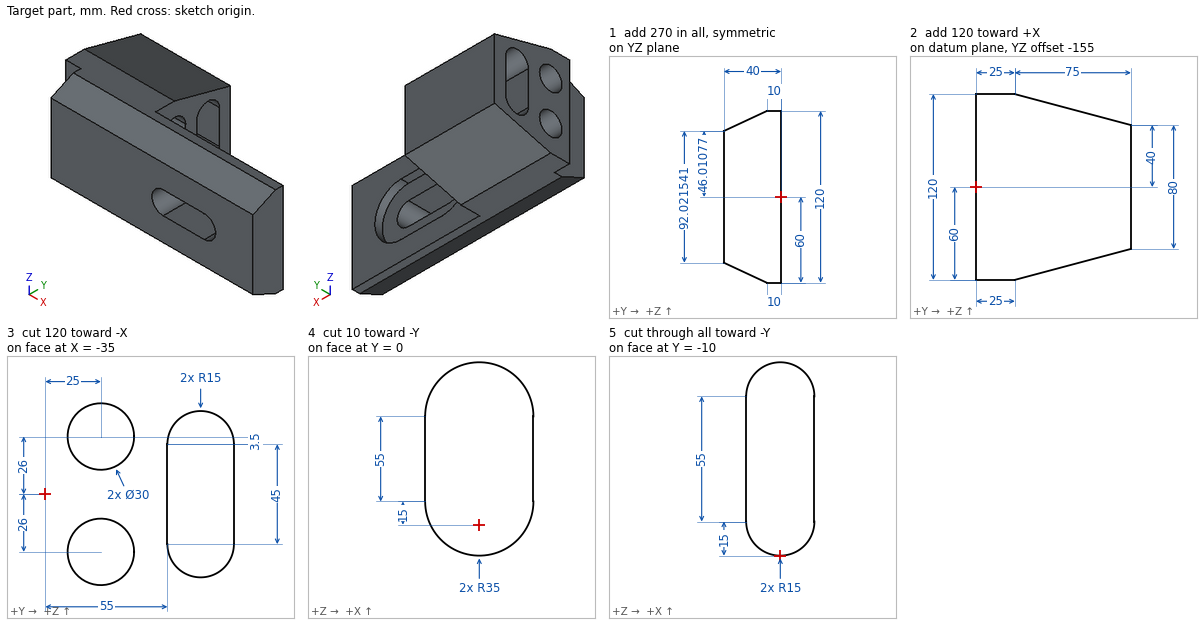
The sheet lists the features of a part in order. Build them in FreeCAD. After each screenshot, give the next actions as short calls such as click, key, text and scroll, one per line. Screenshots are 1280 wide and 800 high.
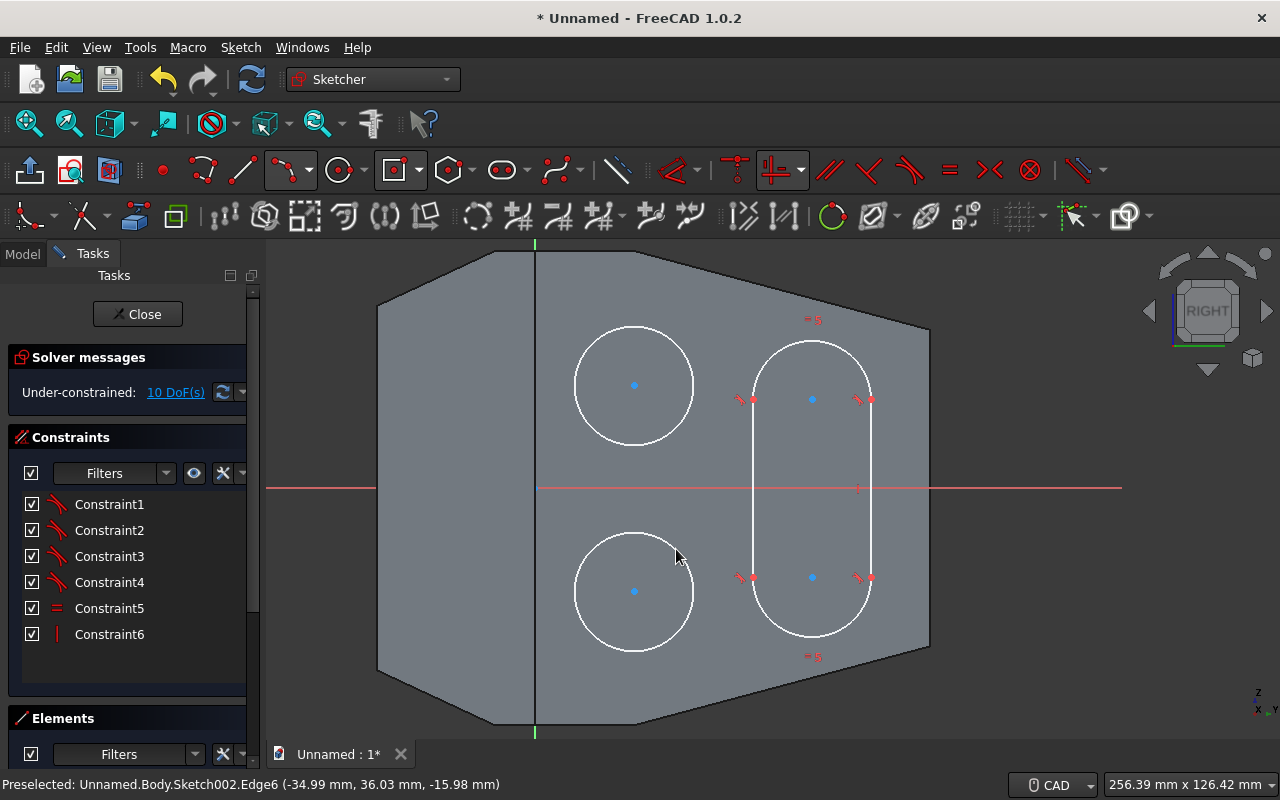
click(676, 344)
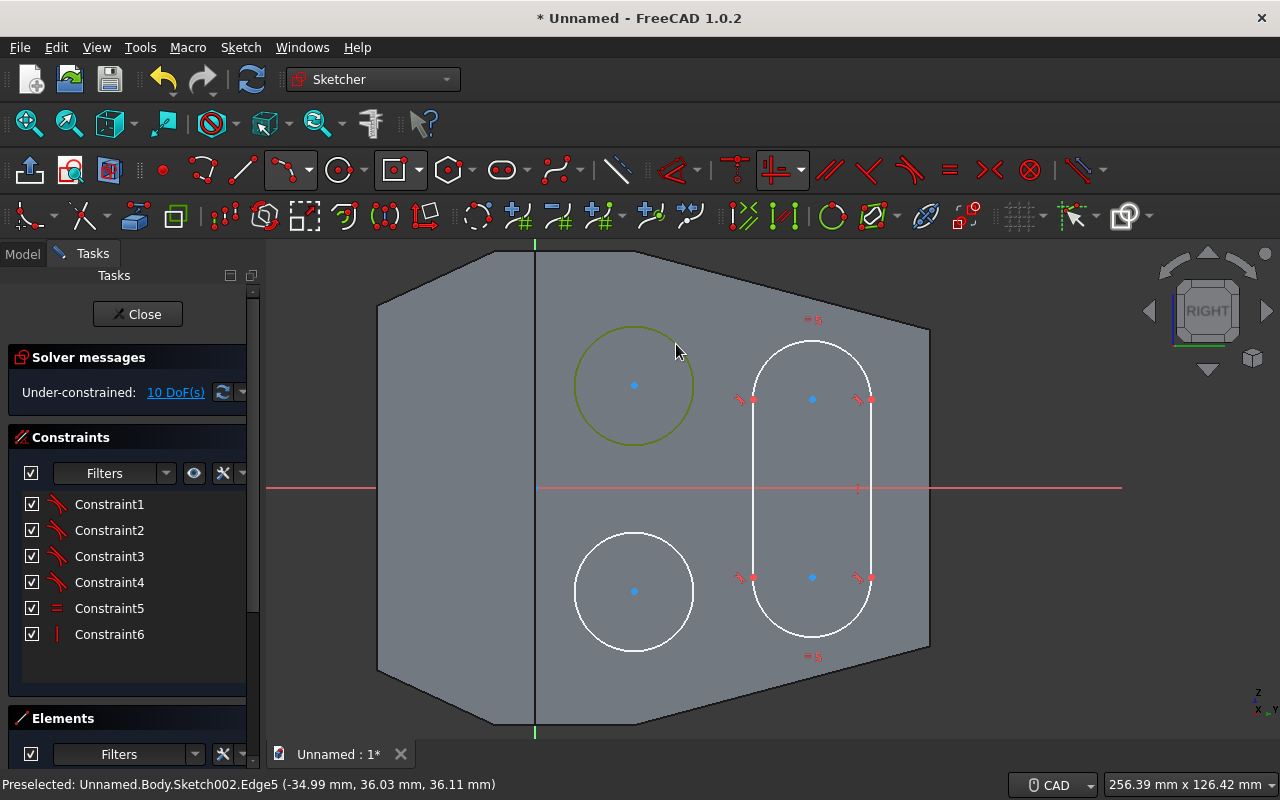
click(676, 550)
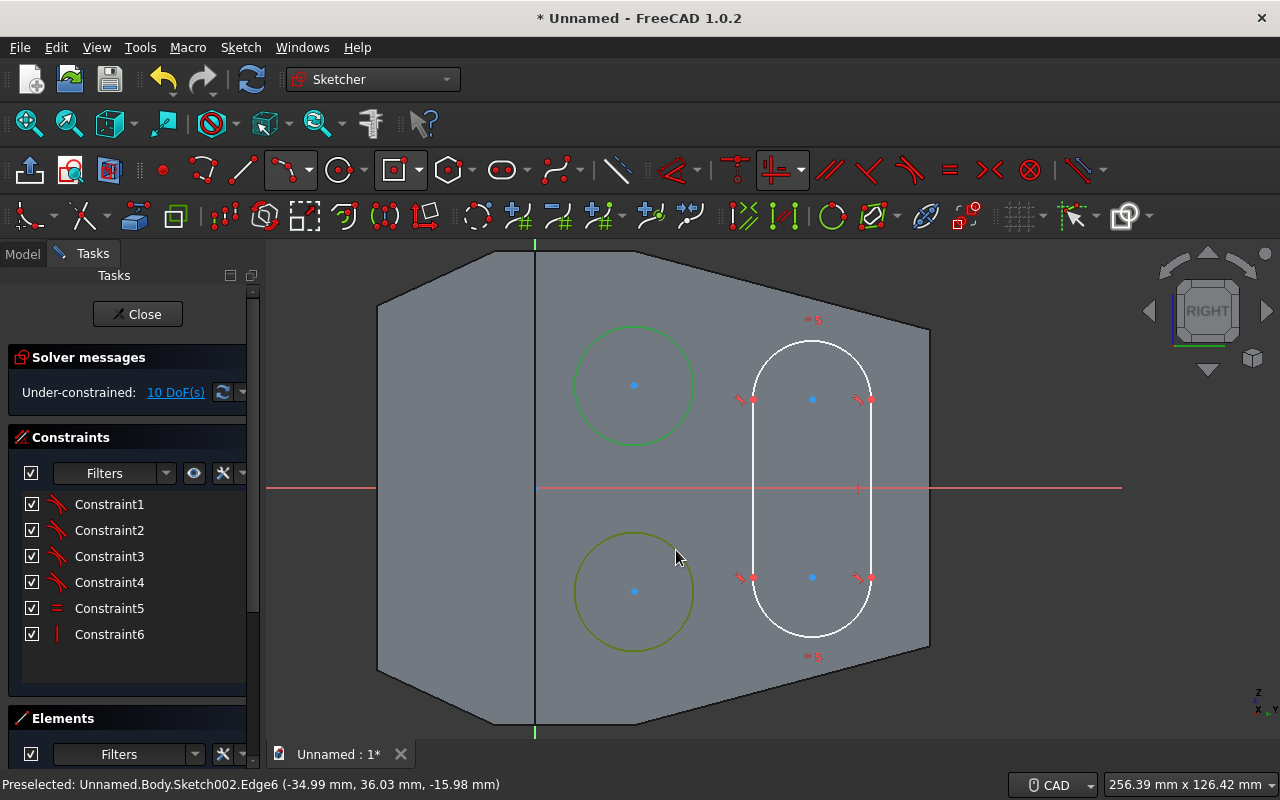
click(950, 170)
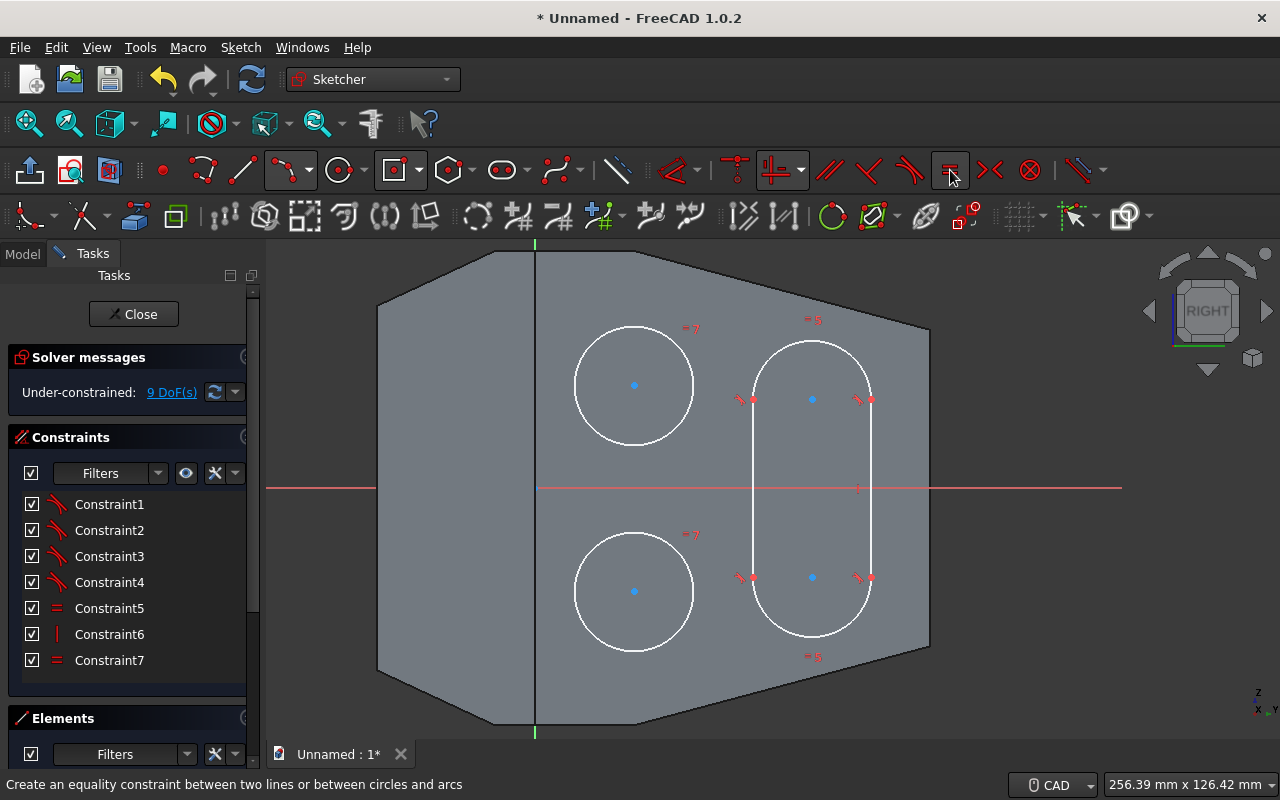
click(634, 386)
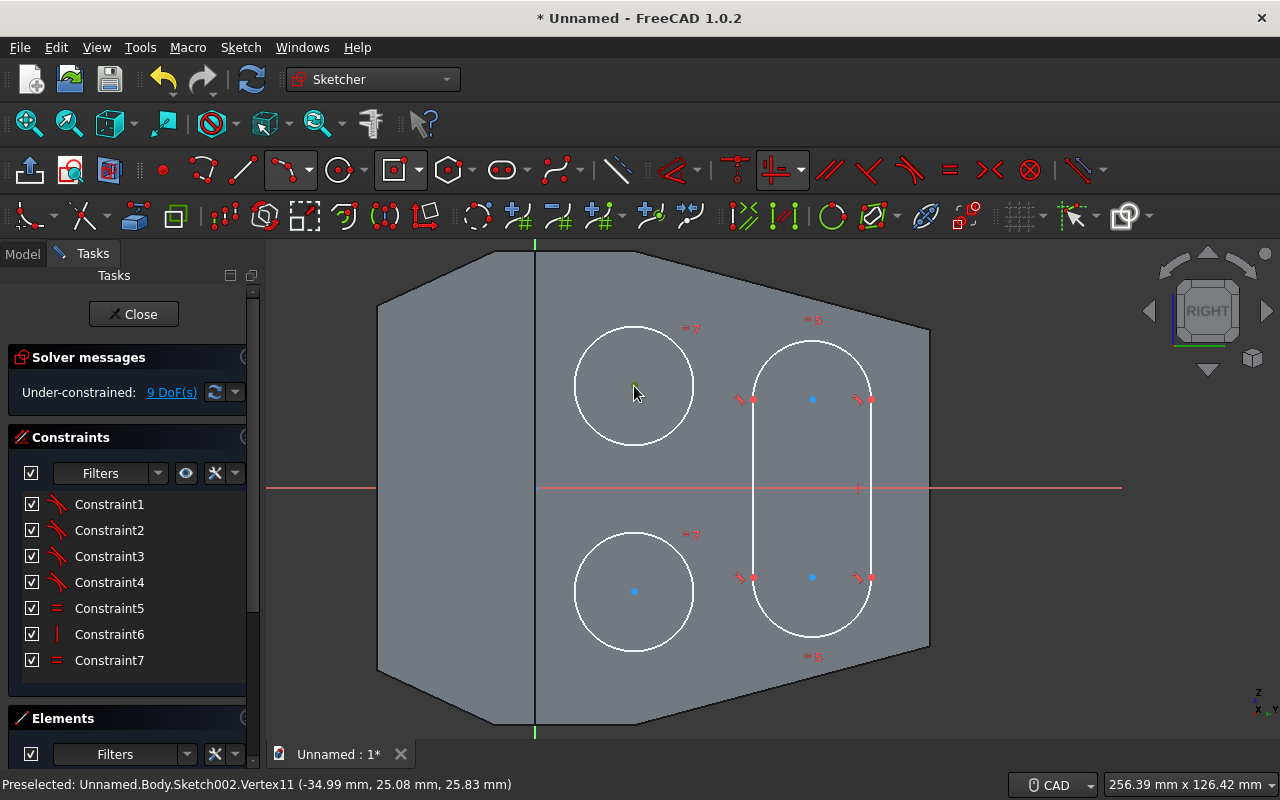
click(634, 592)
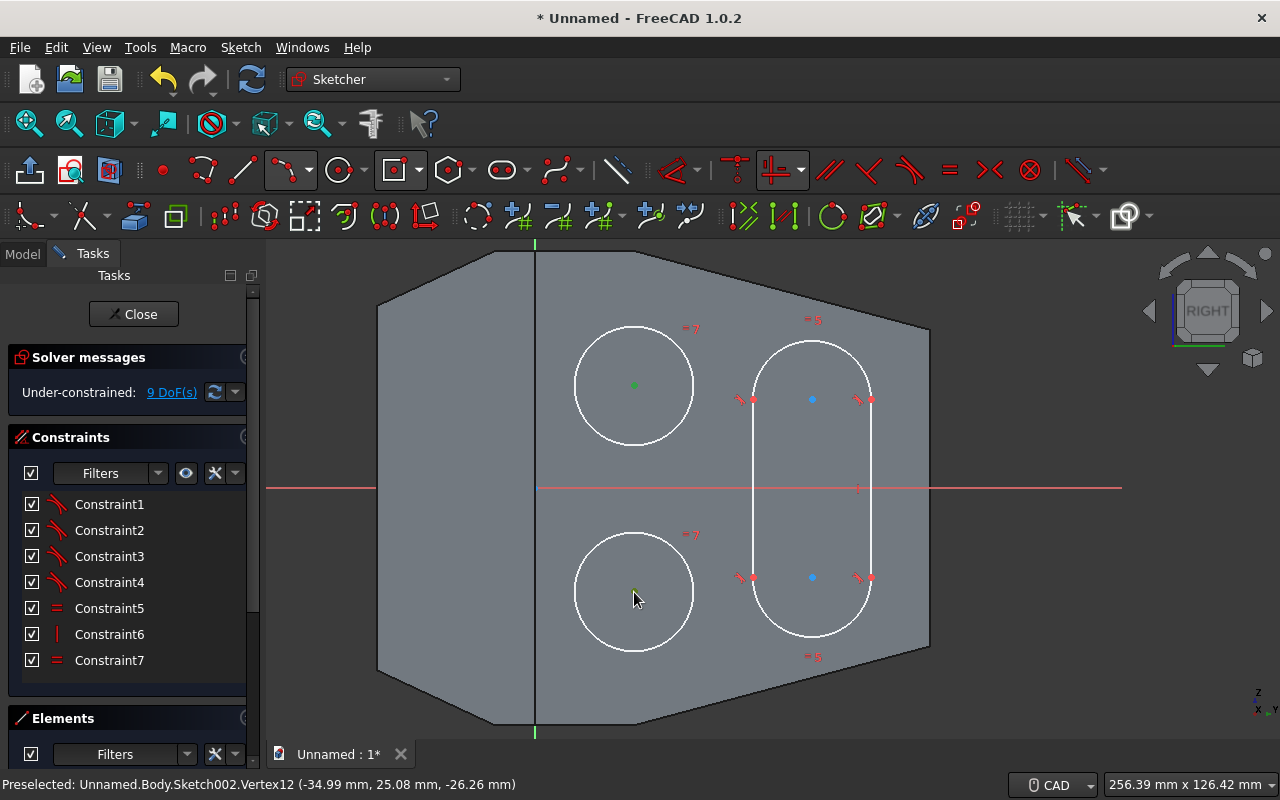
key(v)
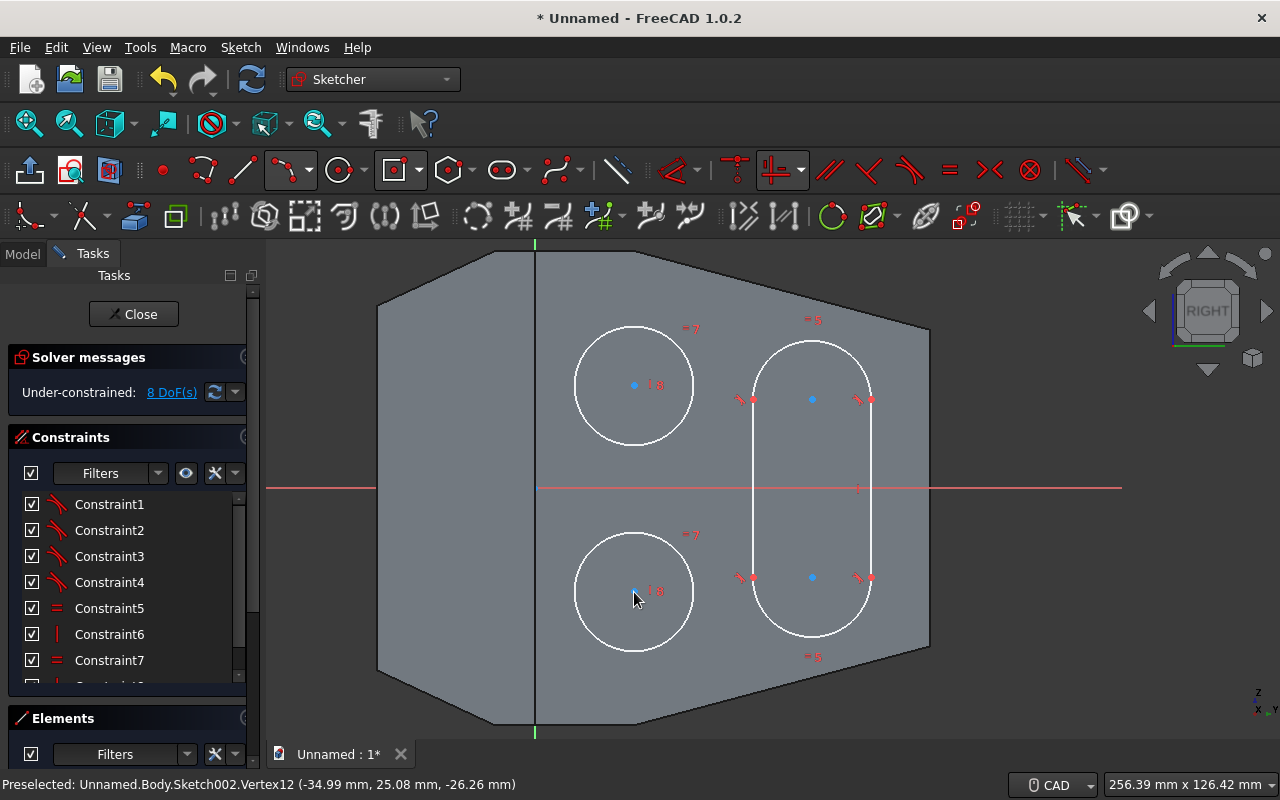
click(672, 170)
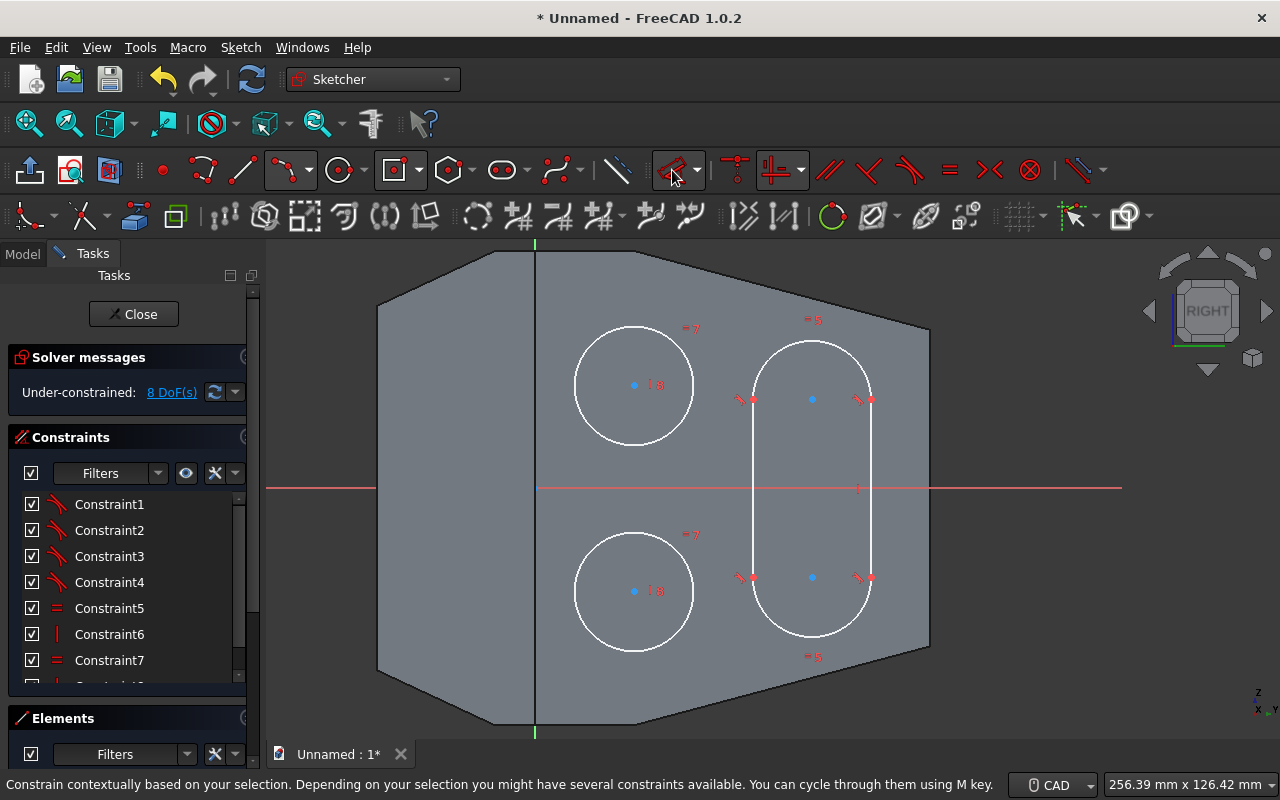
click(777, 626)
click(758, 652)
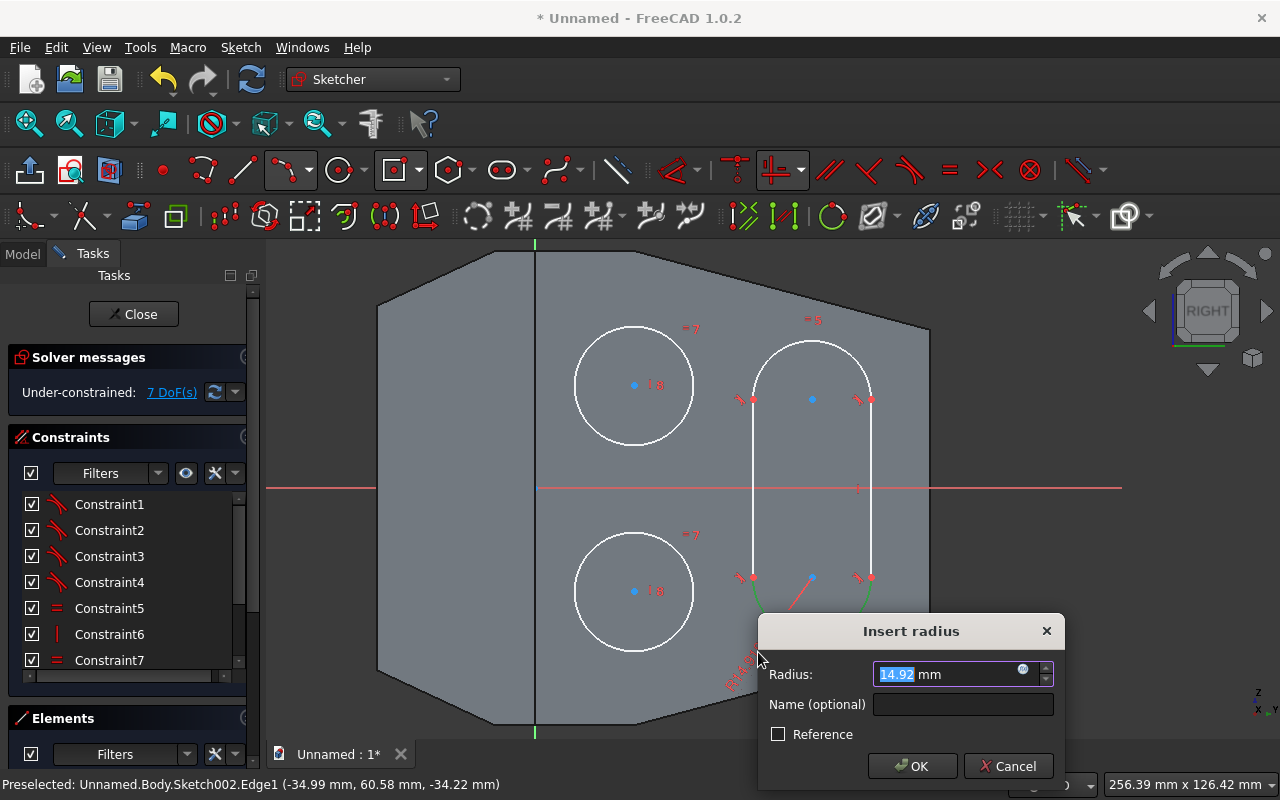
text(15)
key(Return)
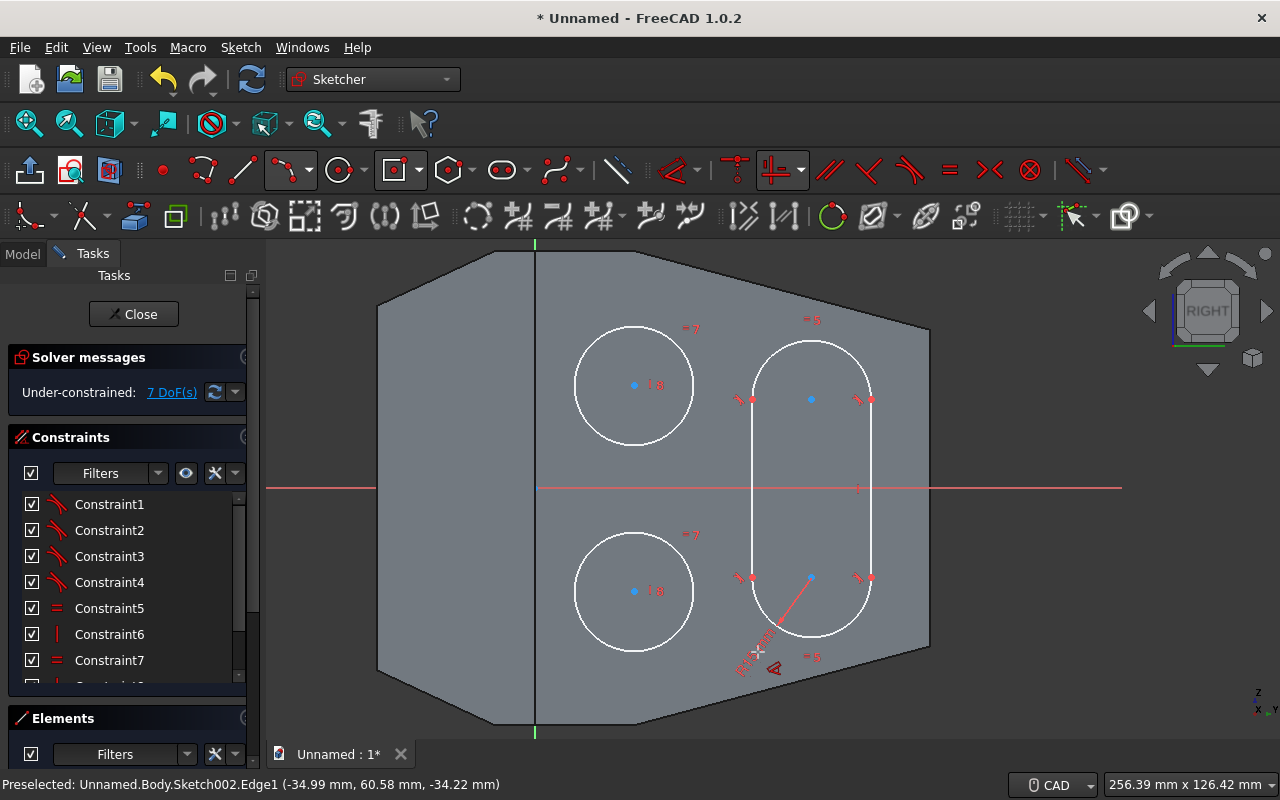
click(676, 344)
click(699, 321)